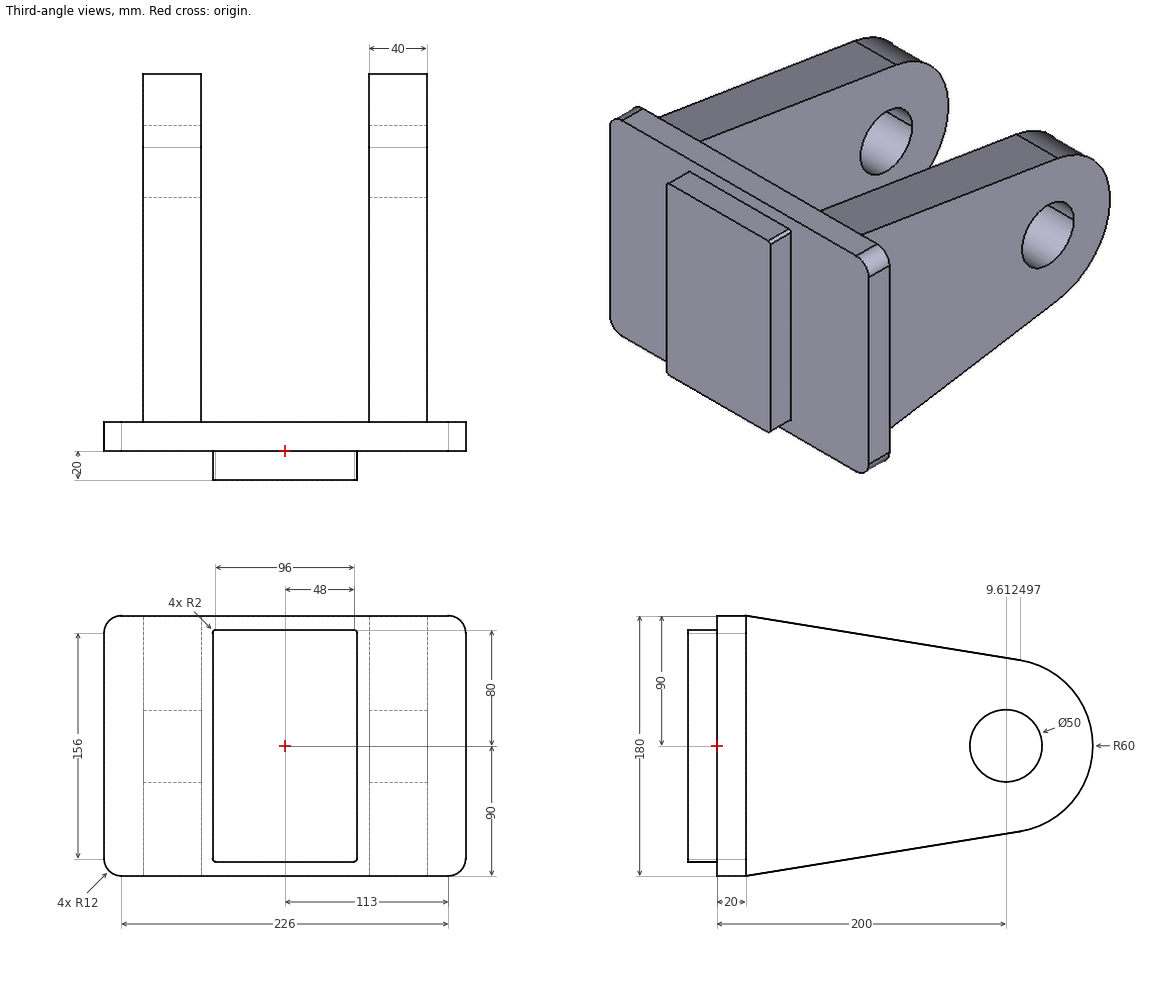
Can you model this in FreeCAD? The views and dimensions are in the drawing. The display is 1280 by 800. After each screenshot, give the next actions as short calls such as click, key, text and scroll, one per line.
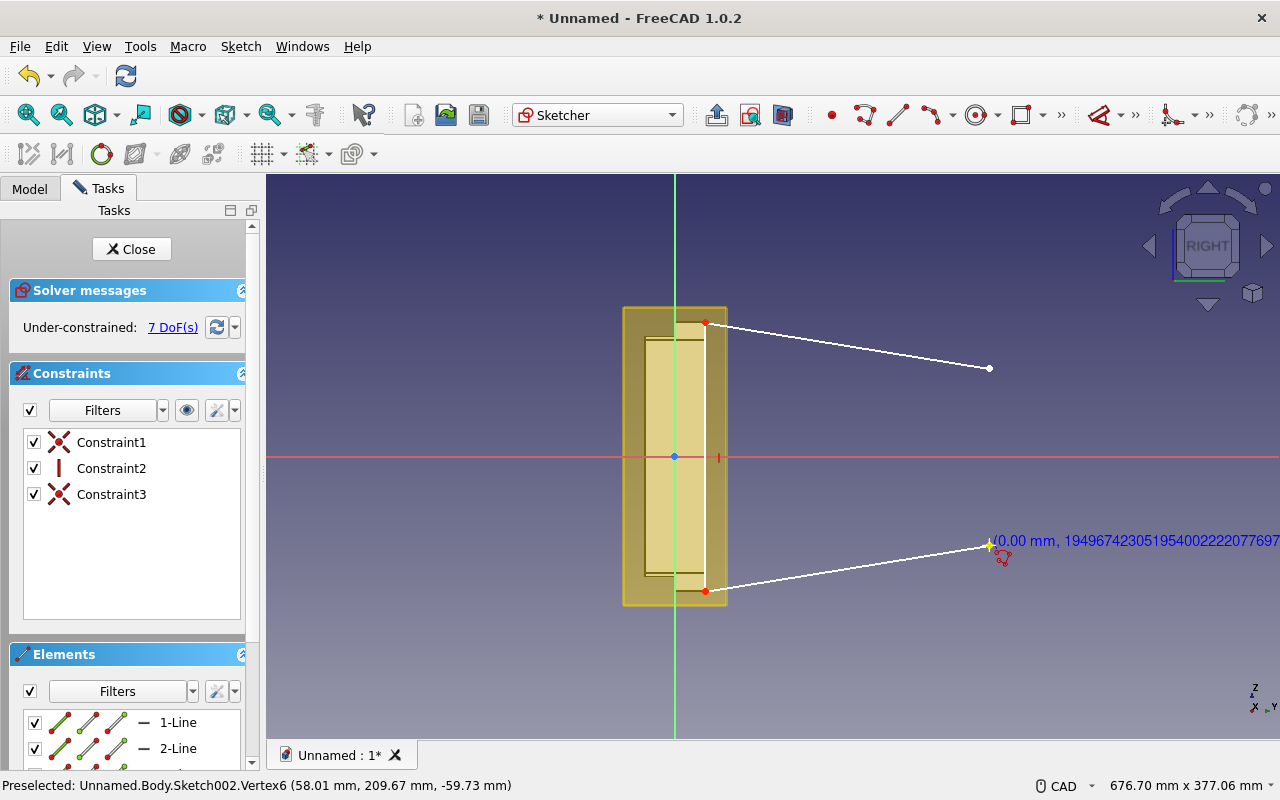
click(930, 116)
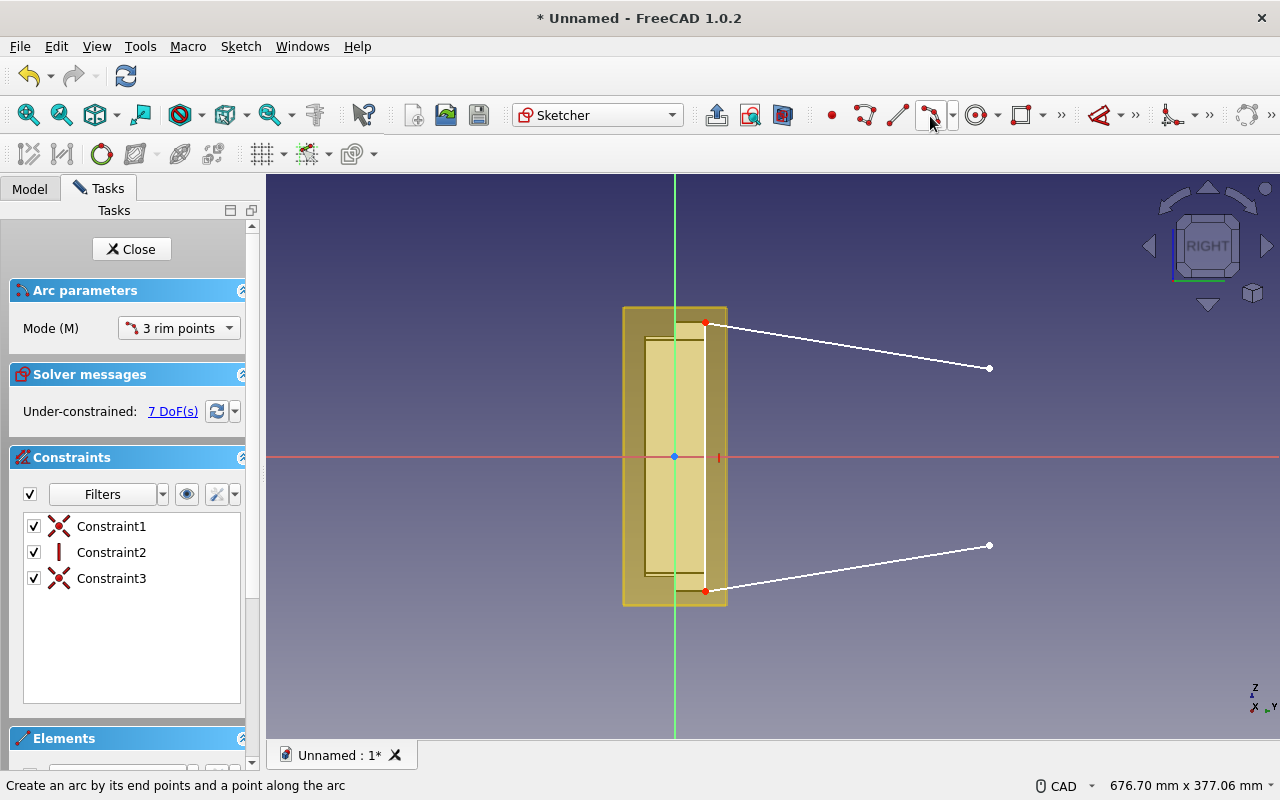
click(989, 546)
click(989, 369)
click(1061, 482)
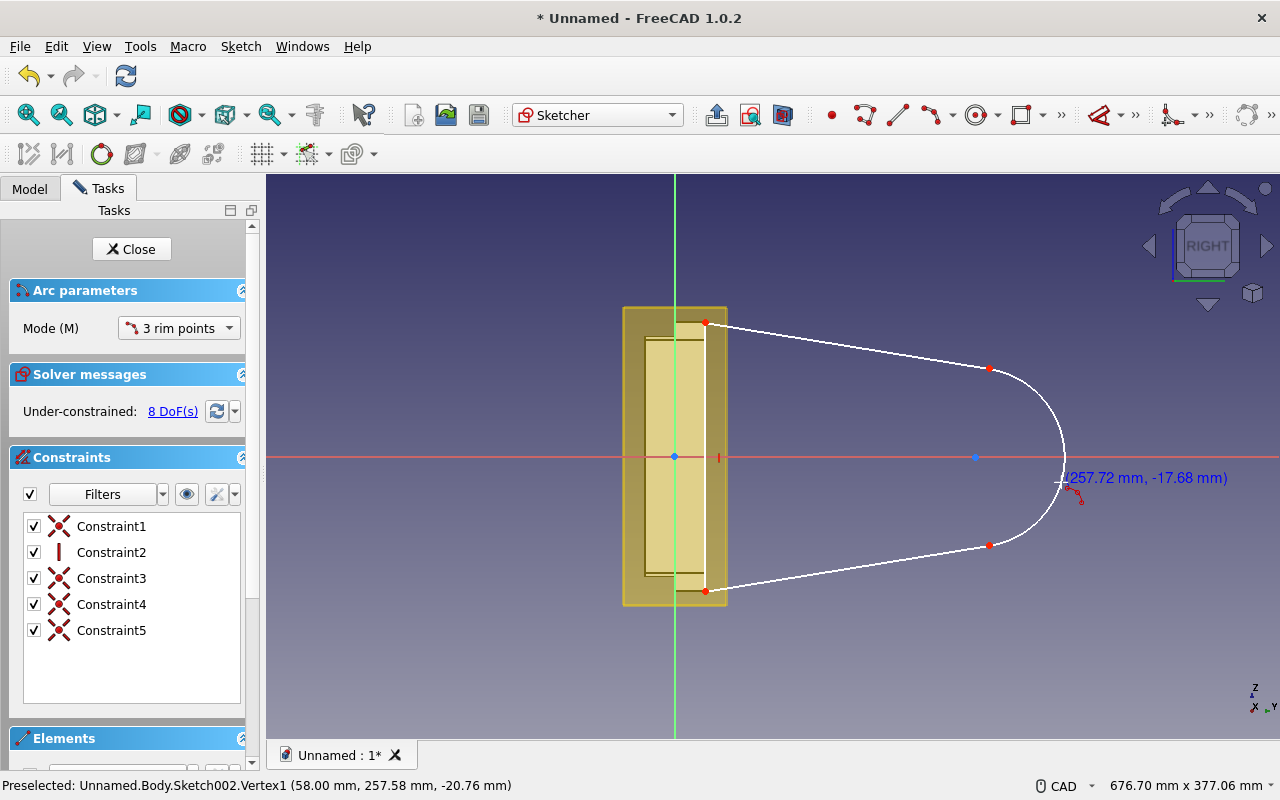
click(976, 116)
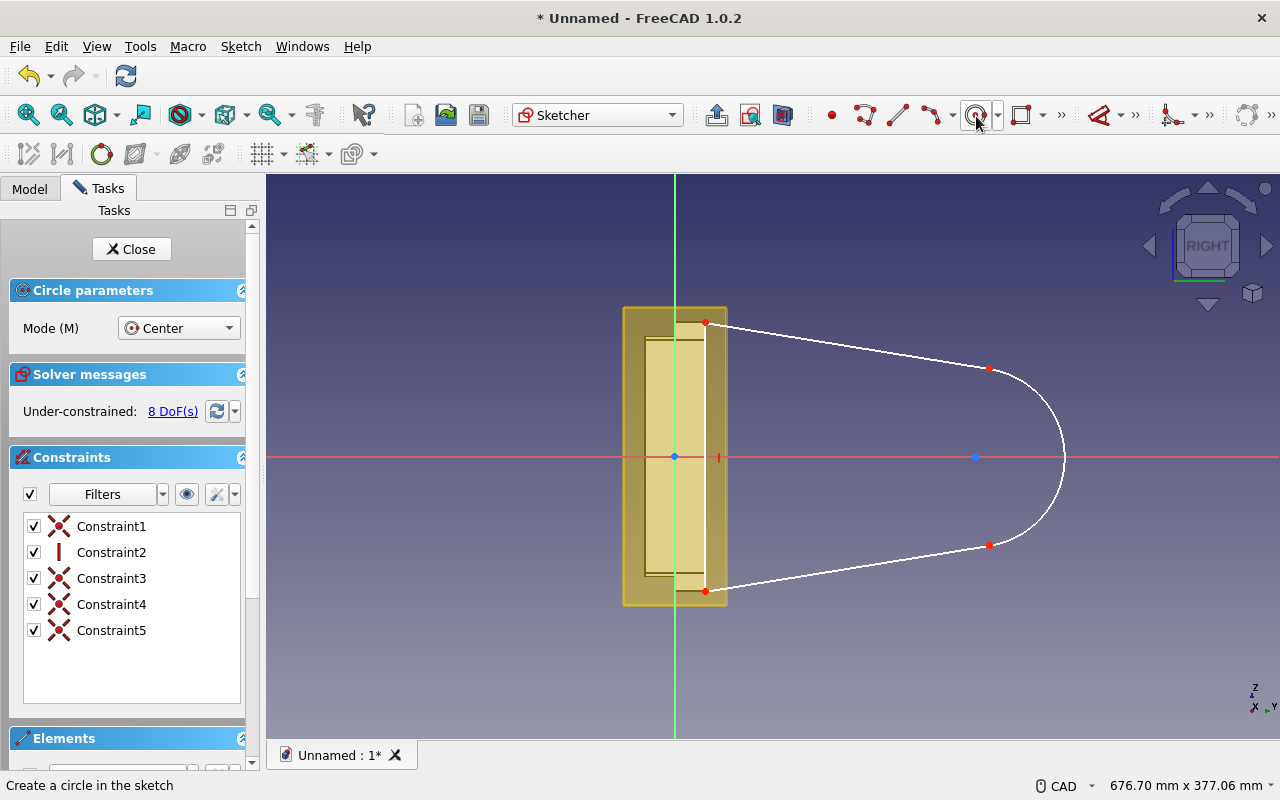
click(975, 457)
click(1001, 430)
key(Escape)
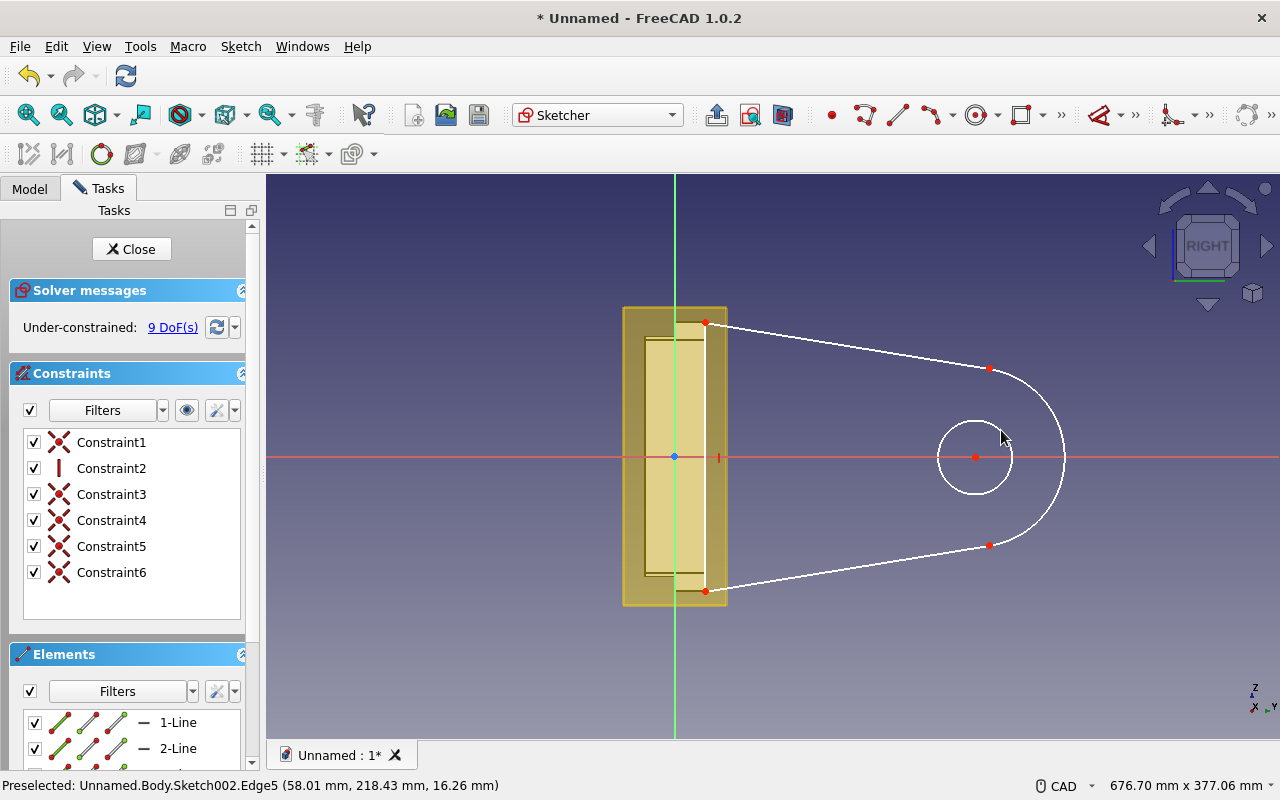
click(975, 458)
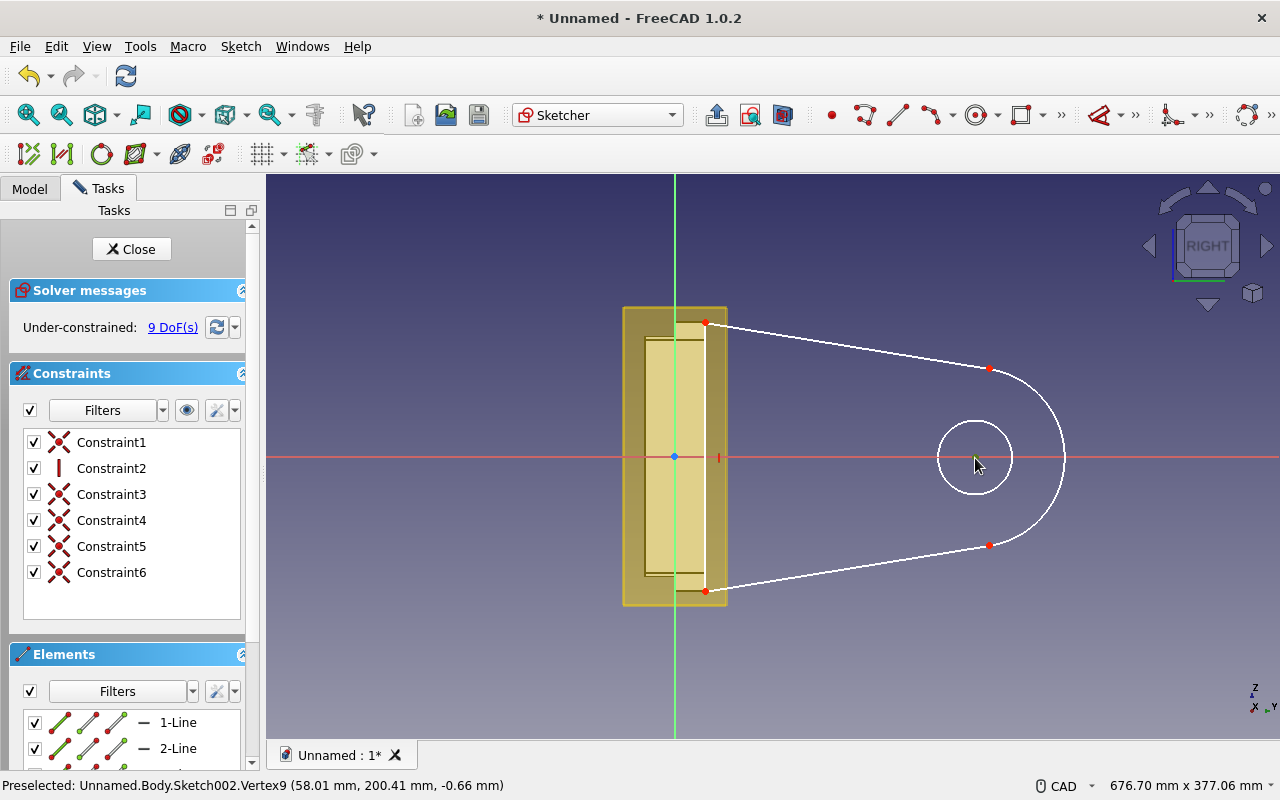
click(353, 457)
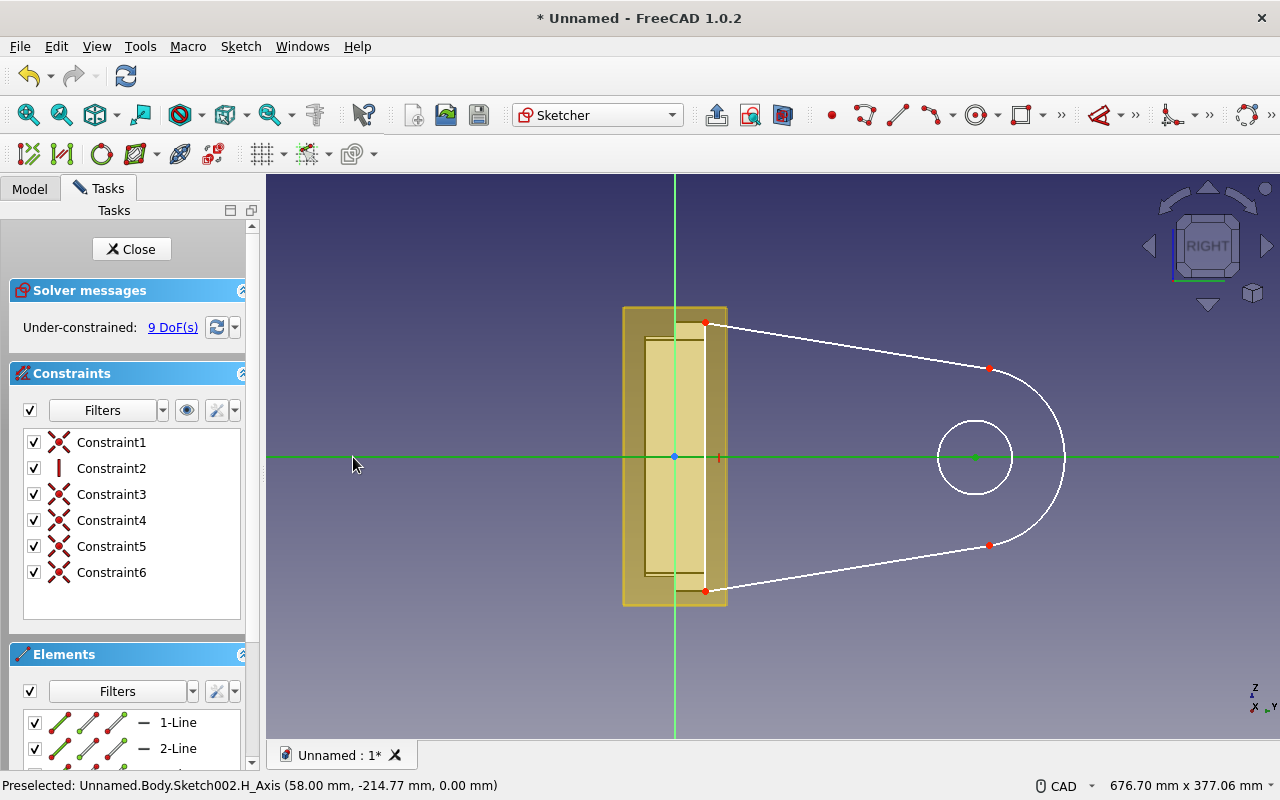
key(c)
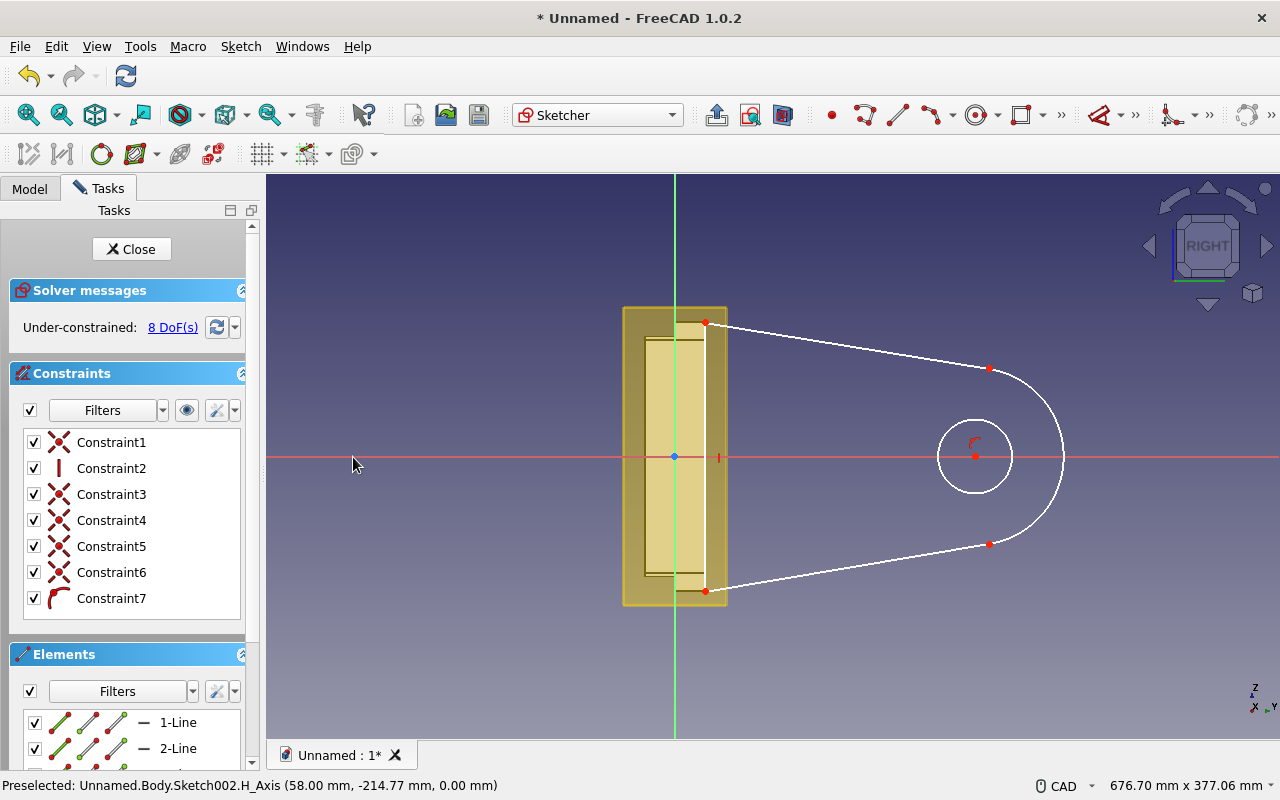
click(1098, 116)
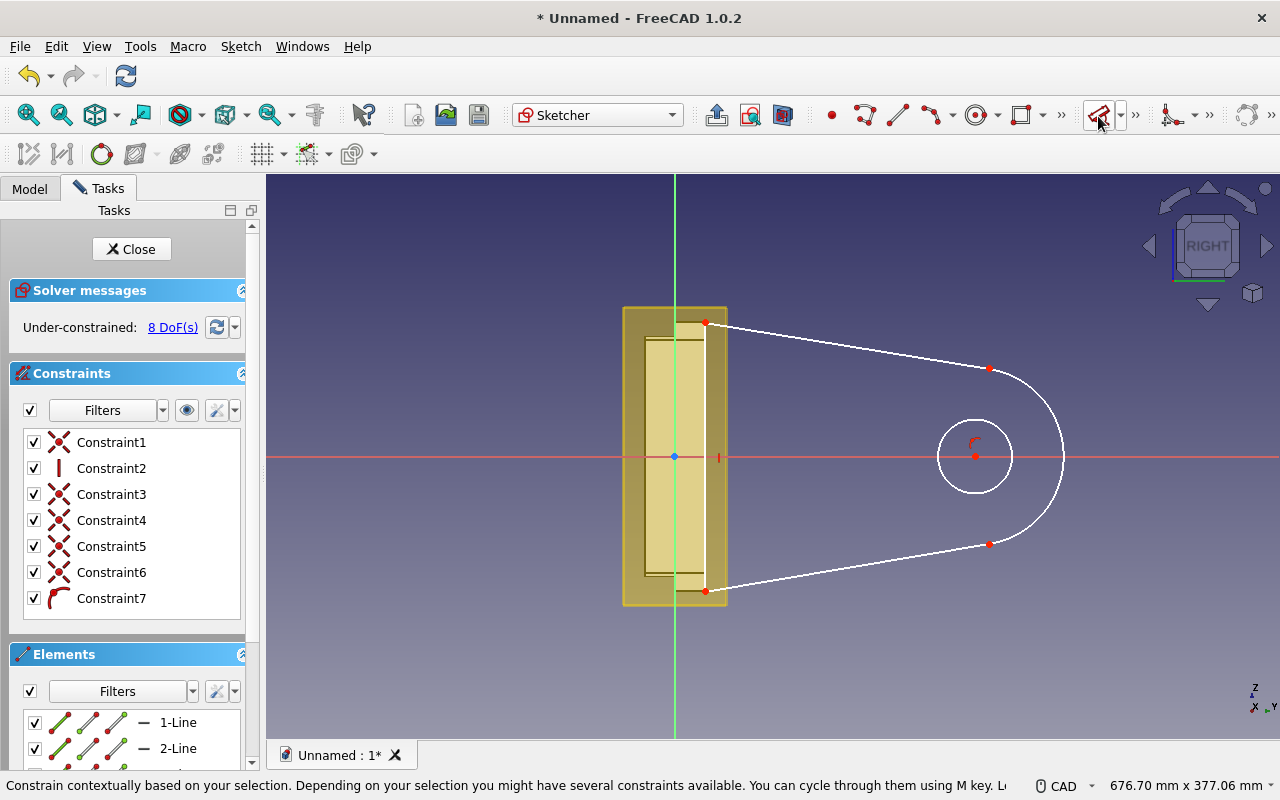
click(1050, 504)
click(1077, 521)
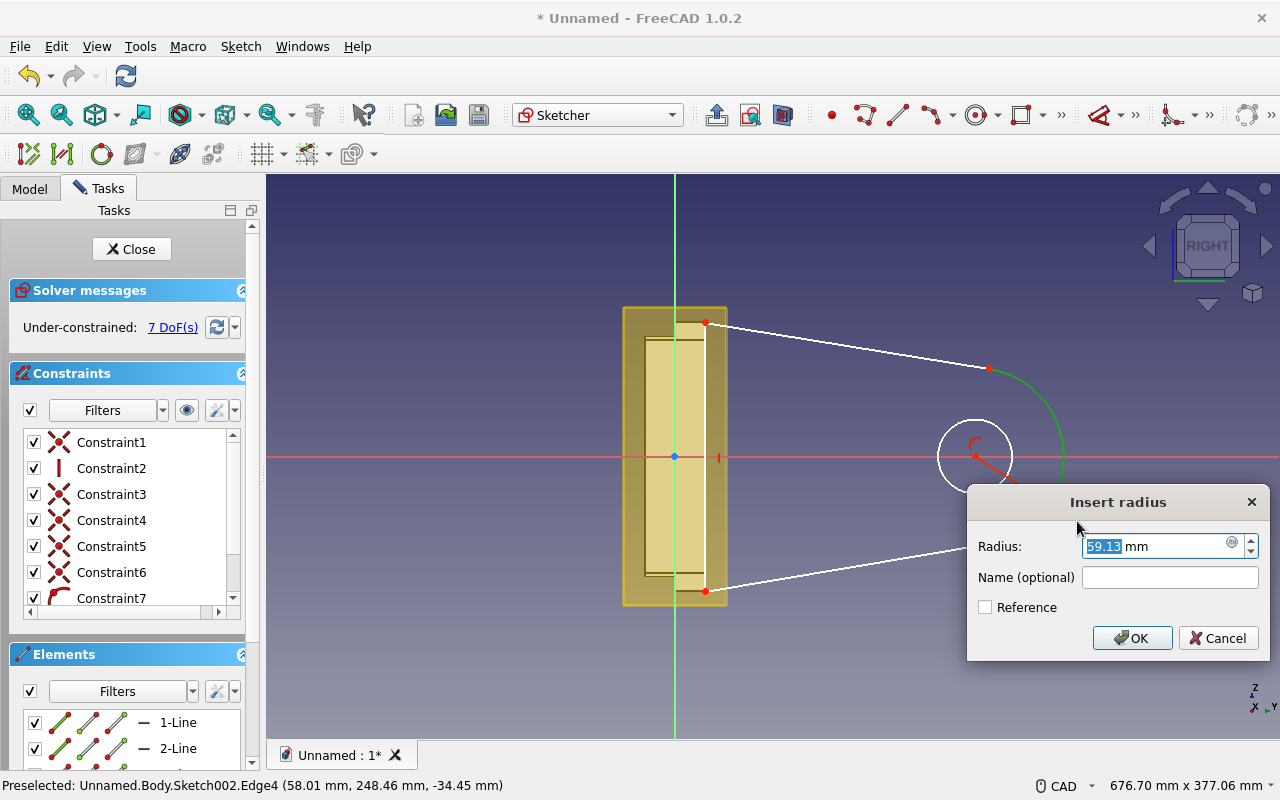
text(60)
key(Return)